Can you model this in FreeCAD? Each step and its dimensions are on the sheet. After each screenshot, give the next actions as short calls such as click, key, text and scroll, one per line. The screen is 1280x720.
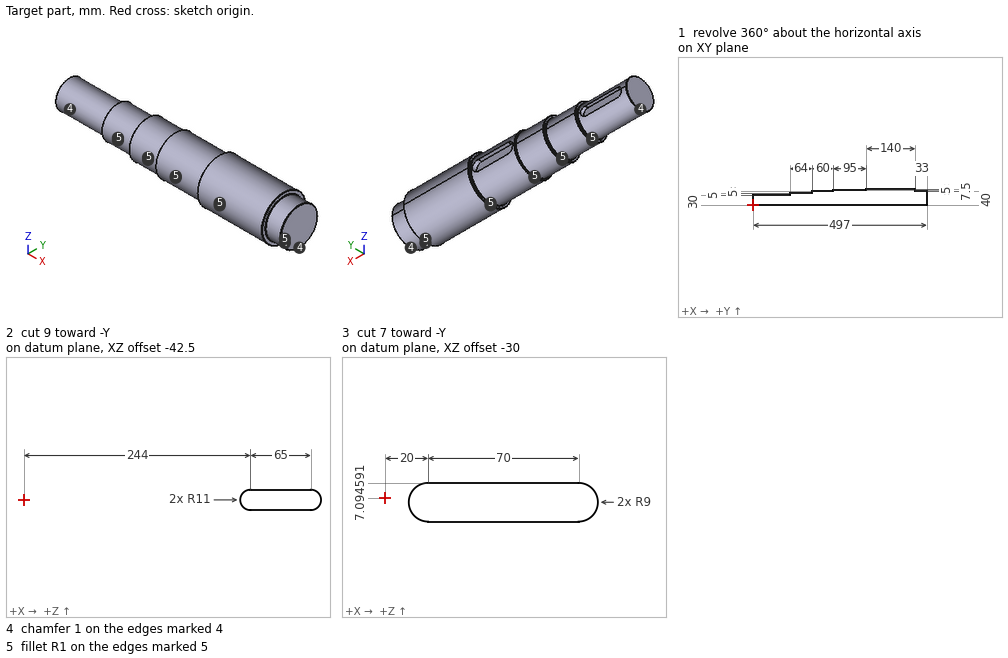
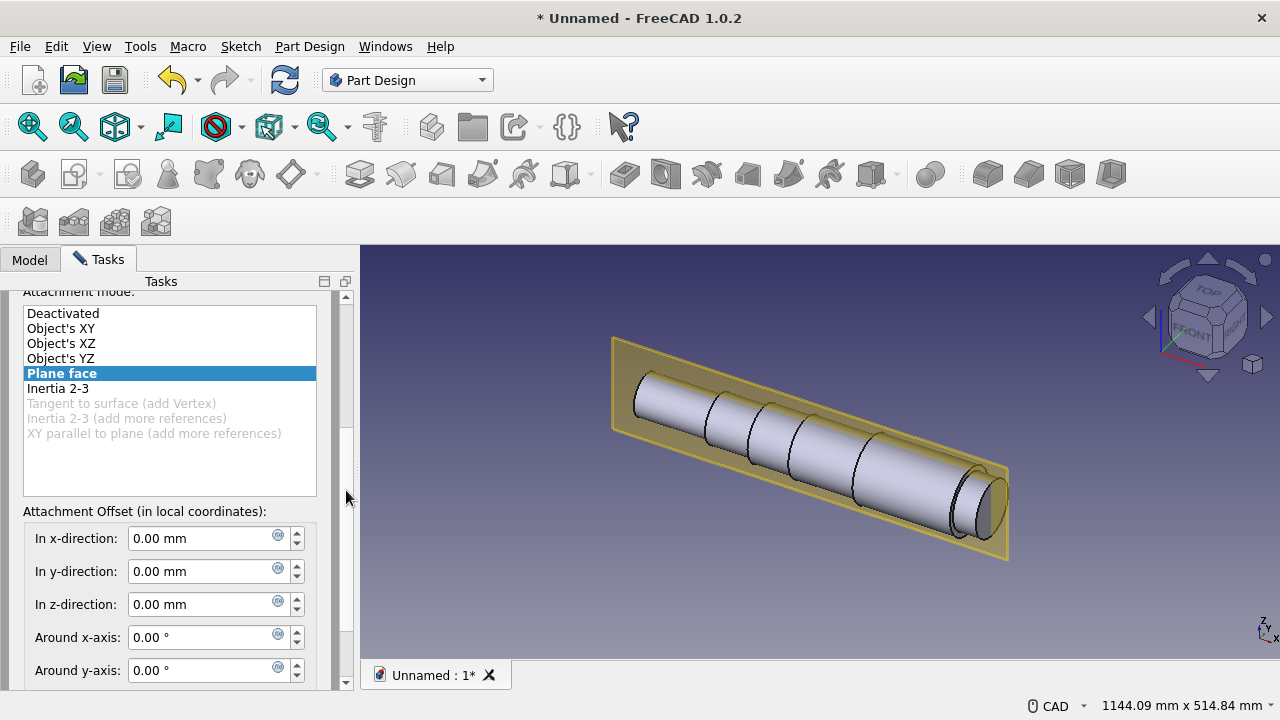
triple_click(210, 604)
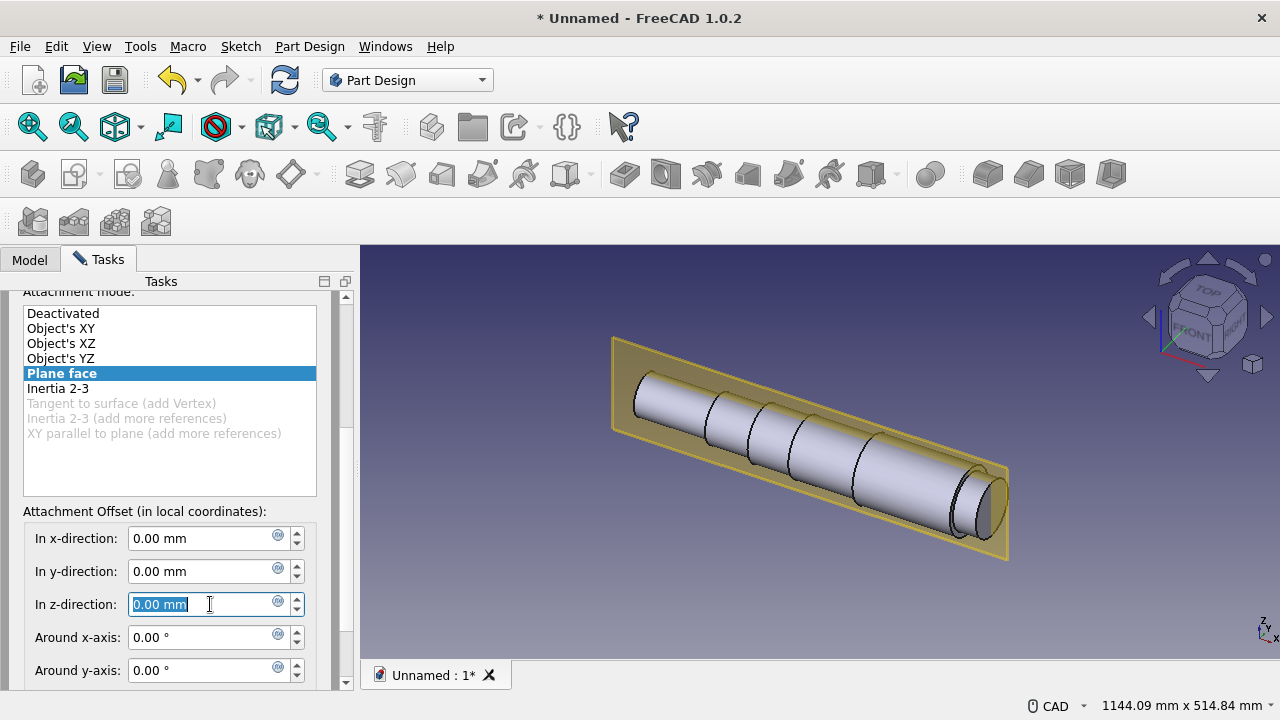
text(-30)
key(Tab)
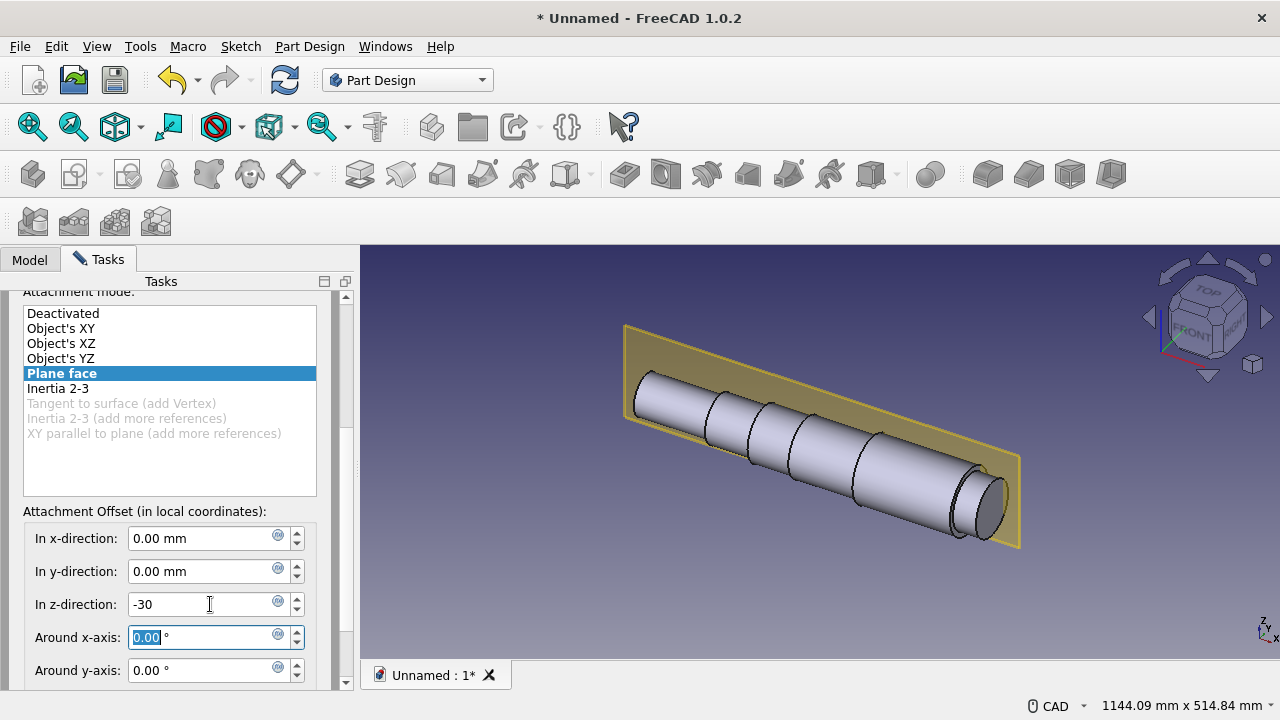
scroll(346, 490, up, 5)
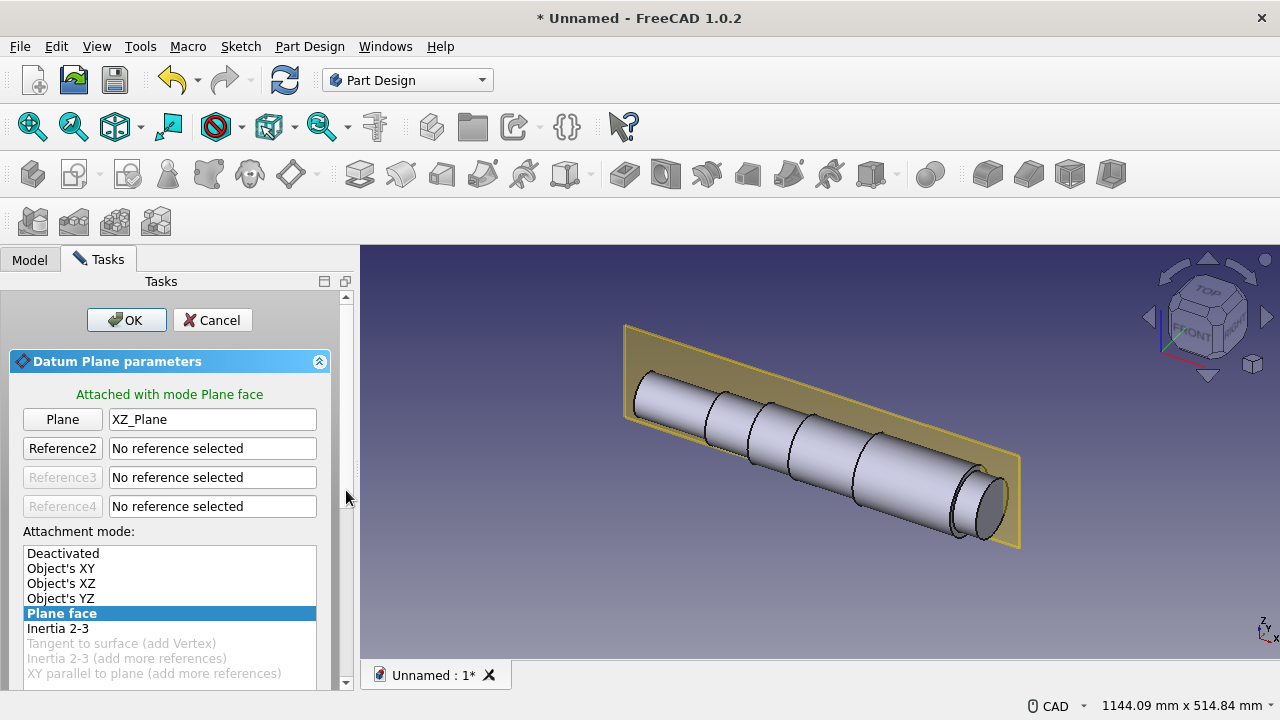
click(127, 320)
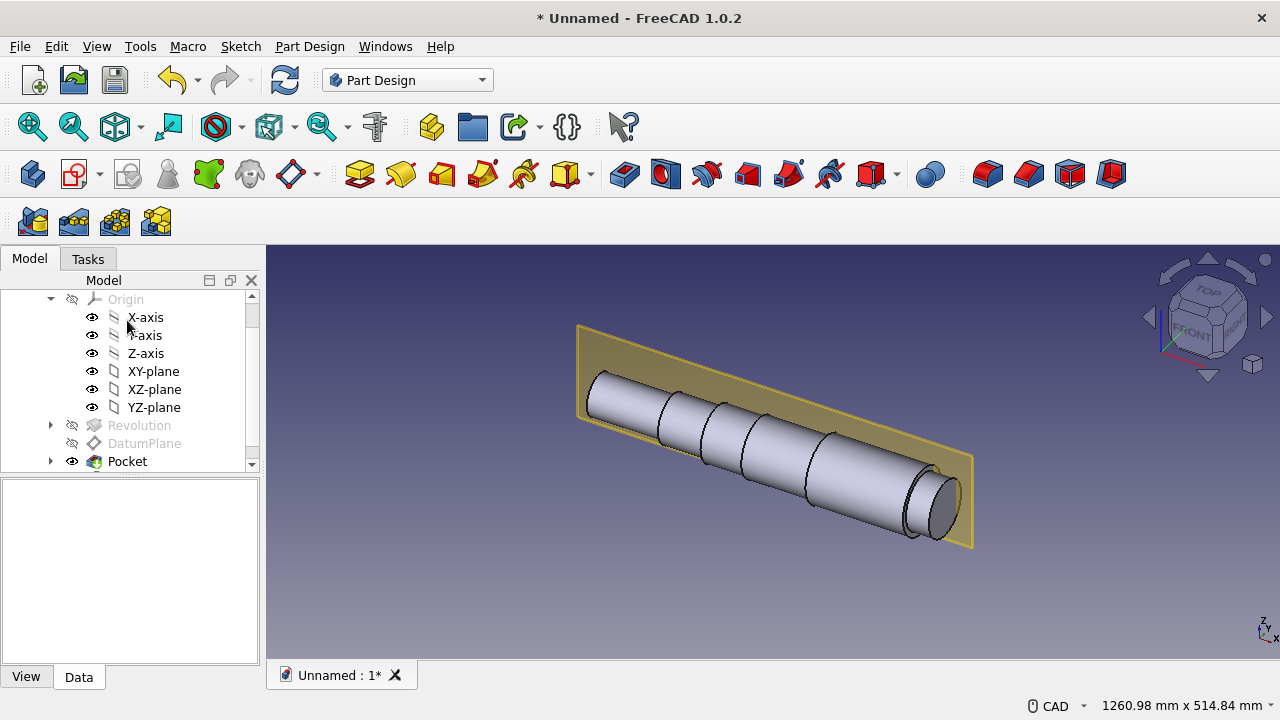
scroll(141, 385, down, 3)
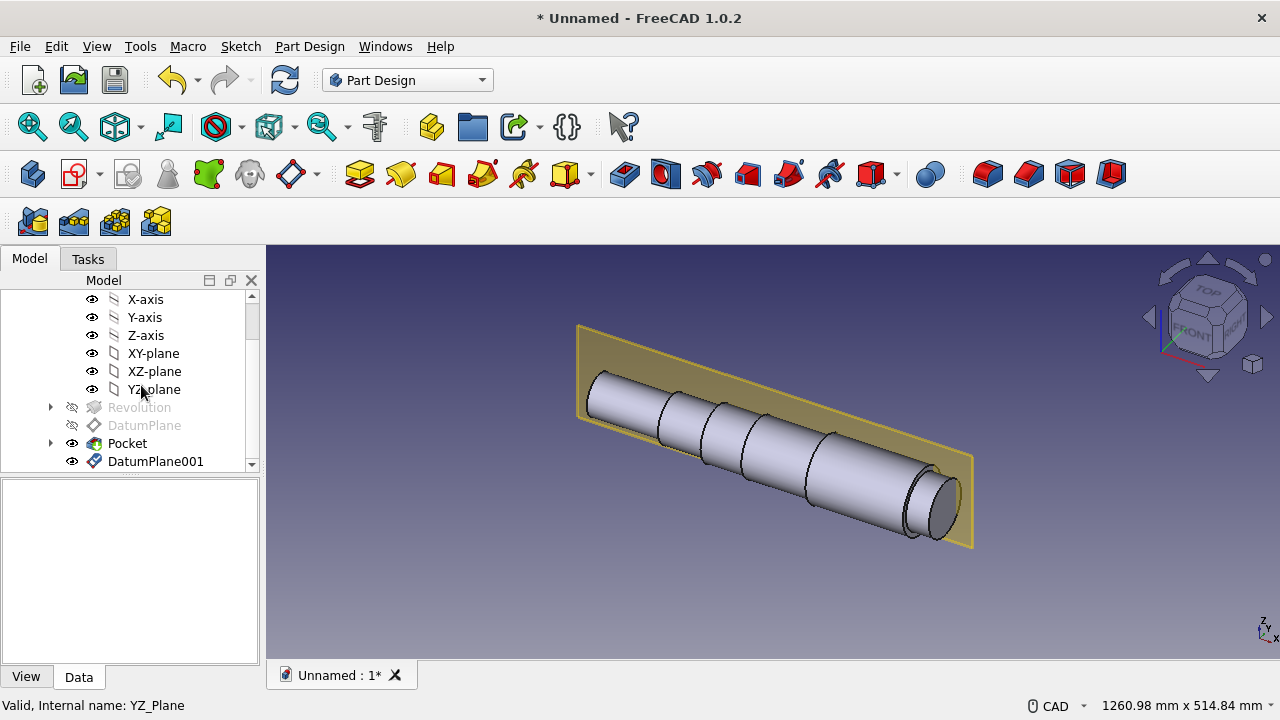
click(117, 461)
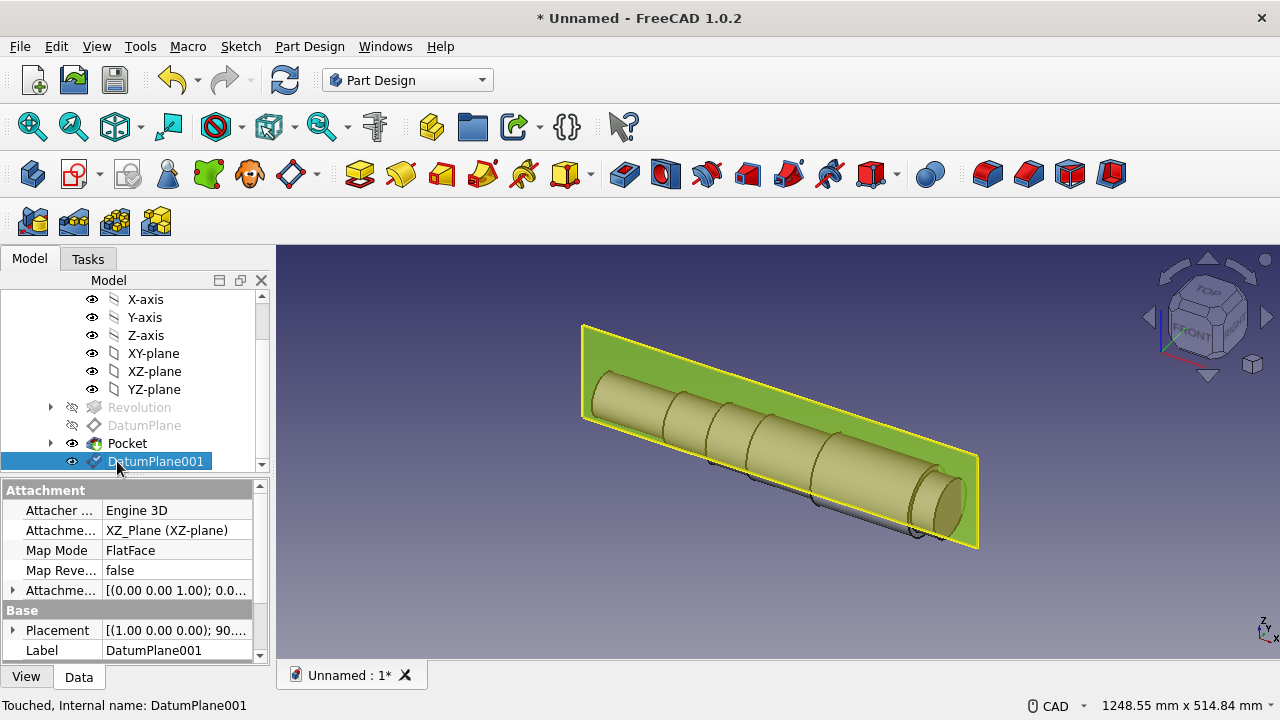
click(74, 174)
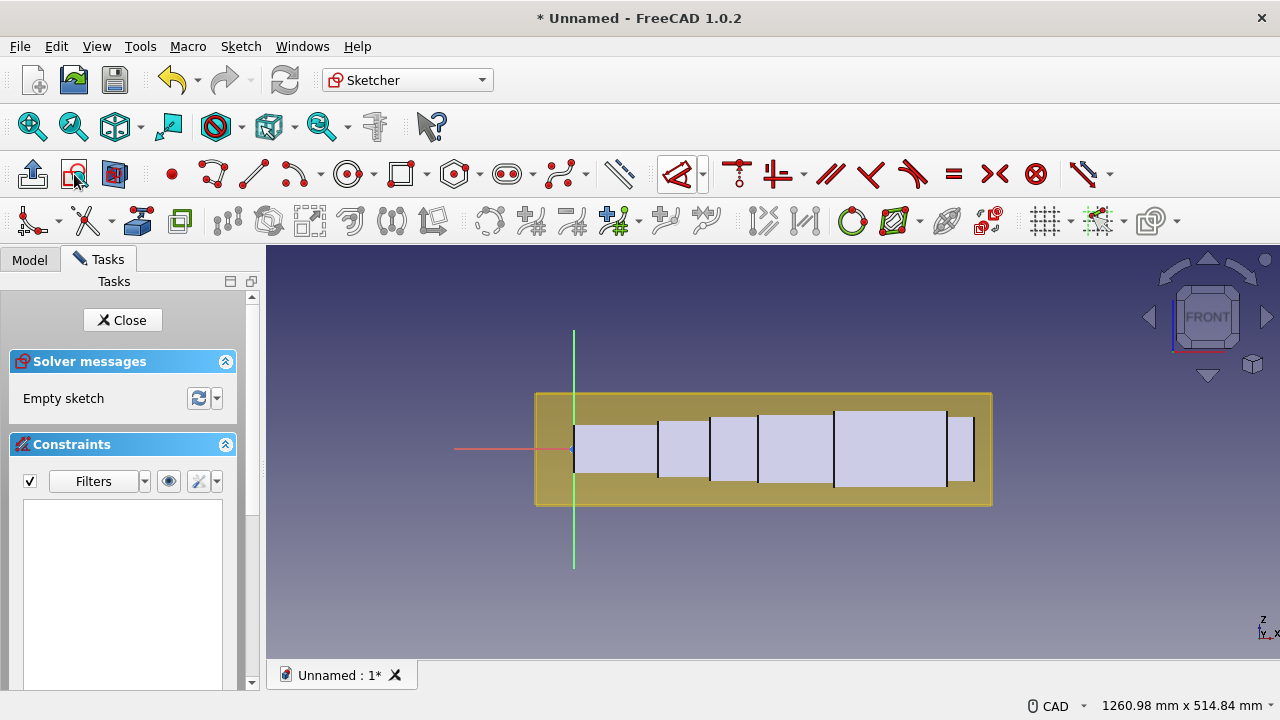
click(115, 174)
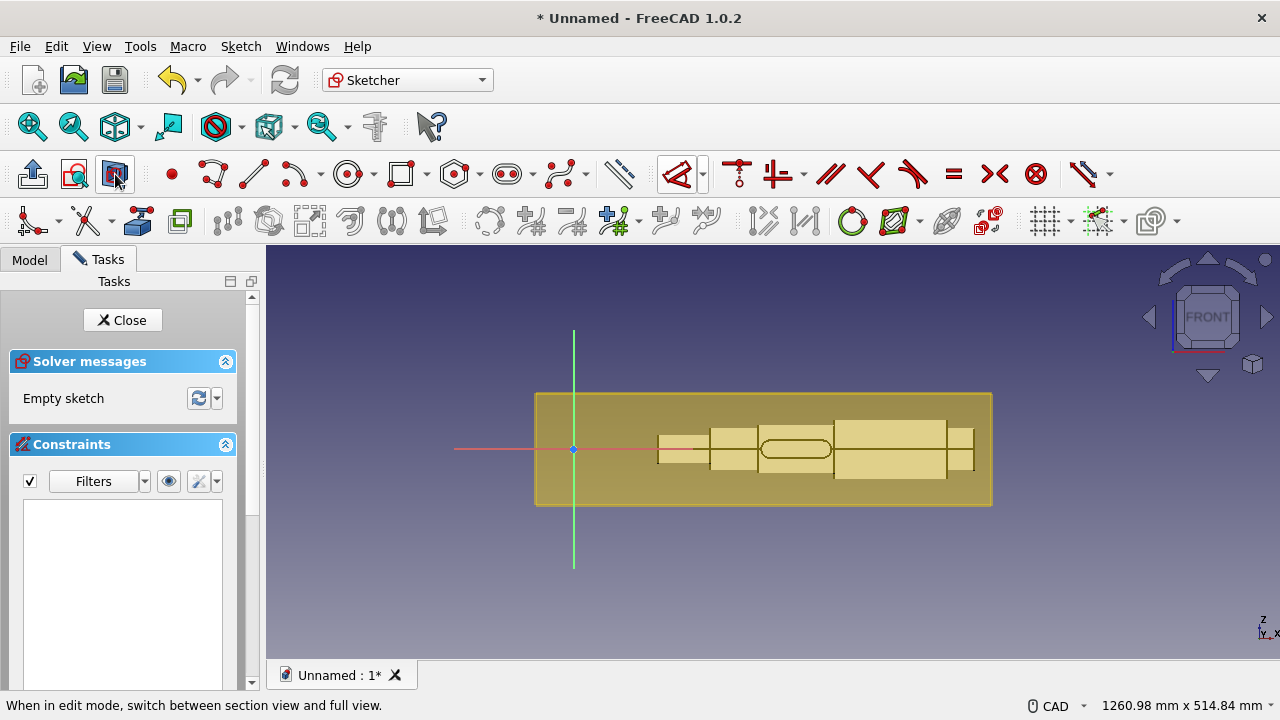
scroll(600, 451, up, 10)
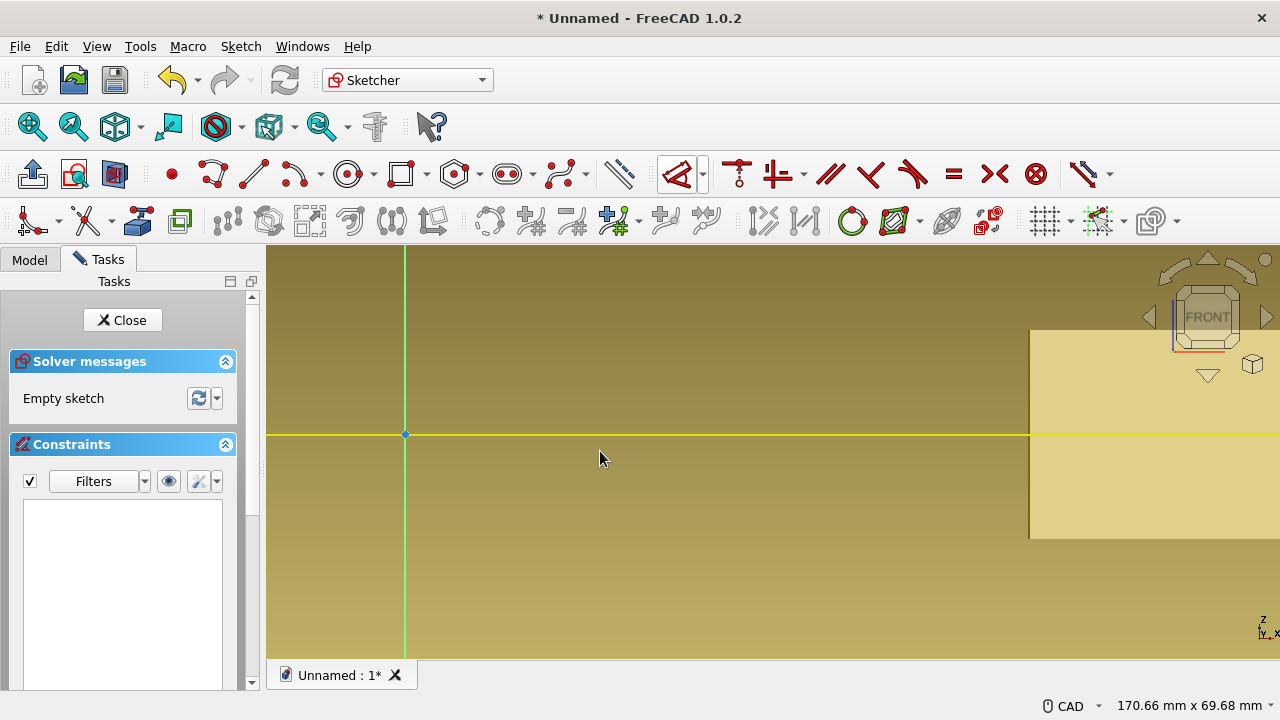
click(506, 174)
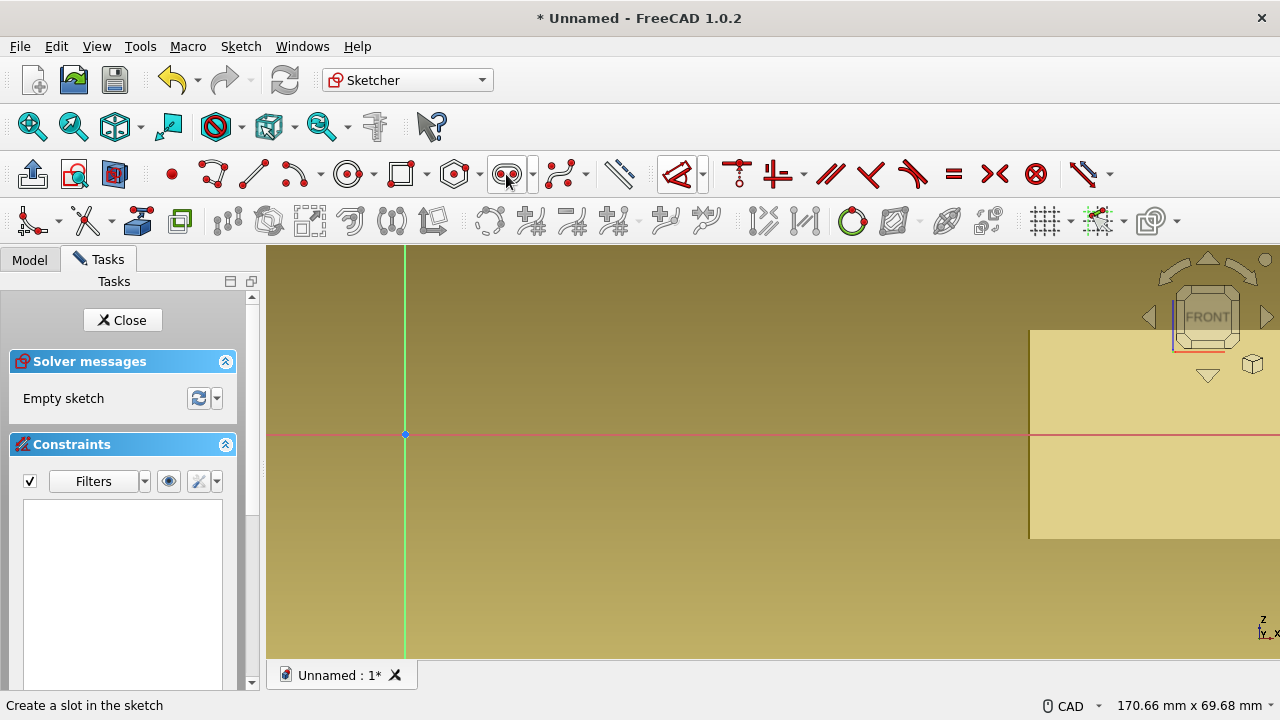
scroll(524, 446, up, 2)